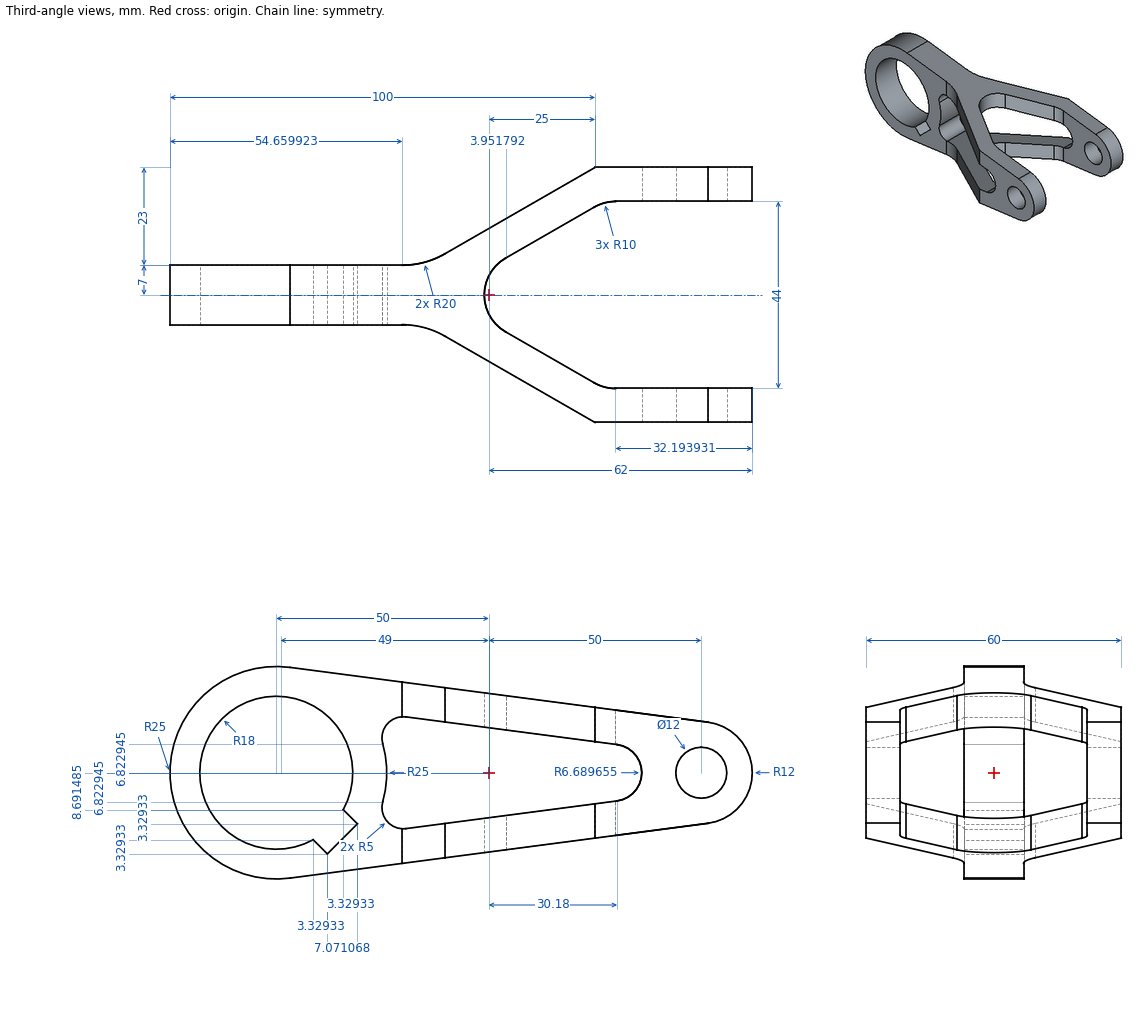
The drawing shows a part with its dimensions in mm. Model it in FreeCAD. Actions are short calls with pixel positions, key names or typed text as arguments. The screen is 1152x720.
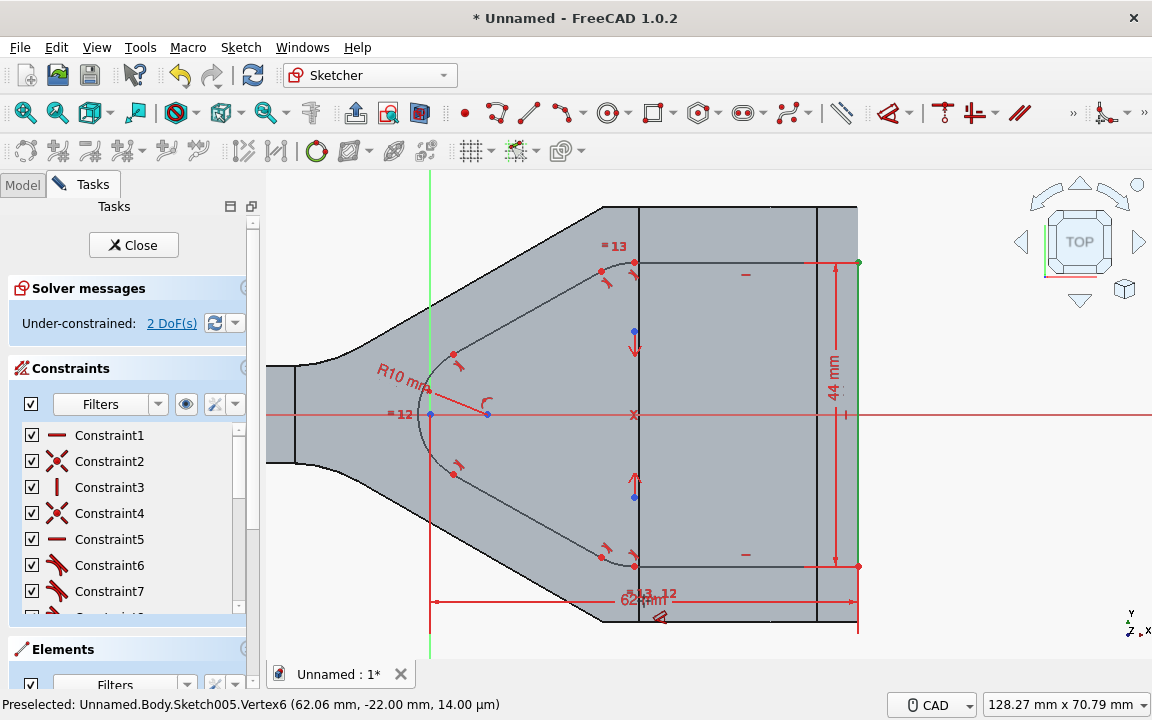
click(702, 567)
click(747, 601)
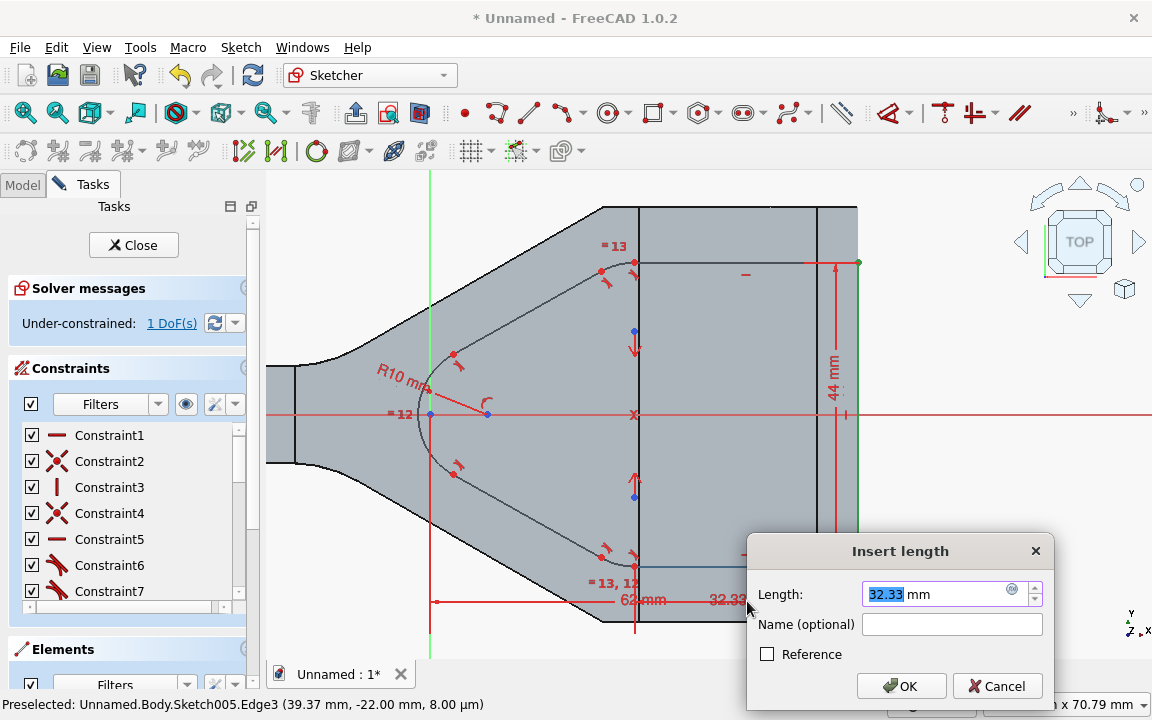
text(32.193931)
key(Return)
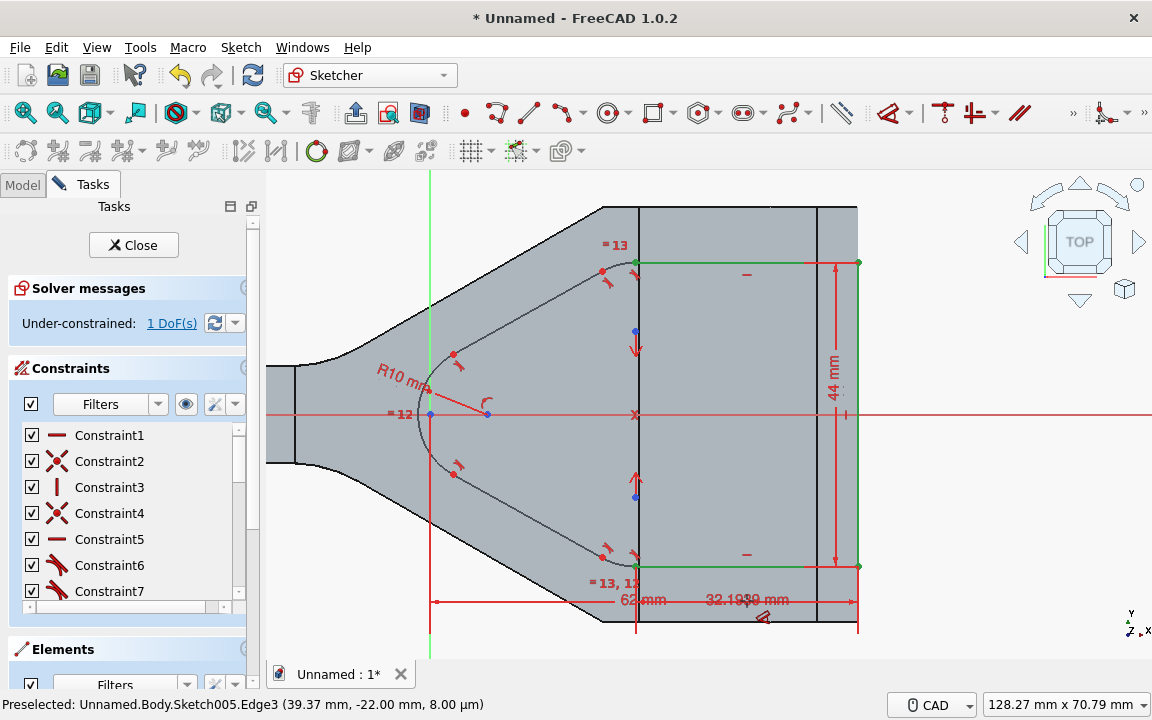
scroll(454, 354, up, 2)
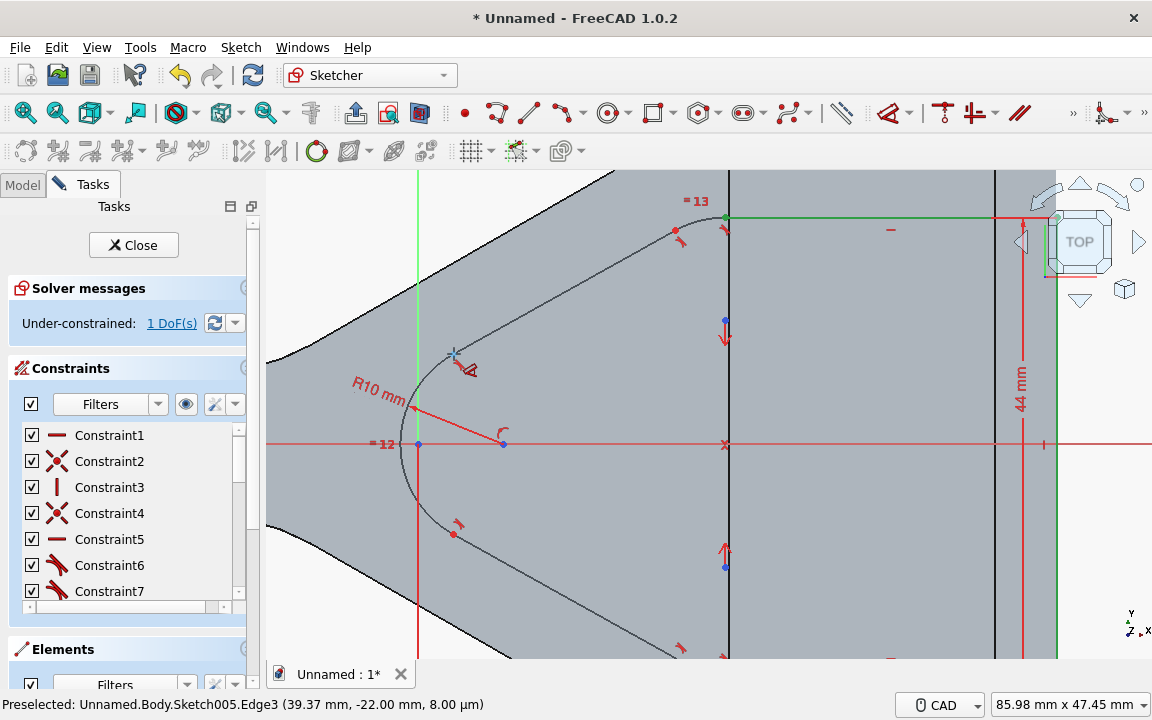
click(453, 354)
click(436, 320)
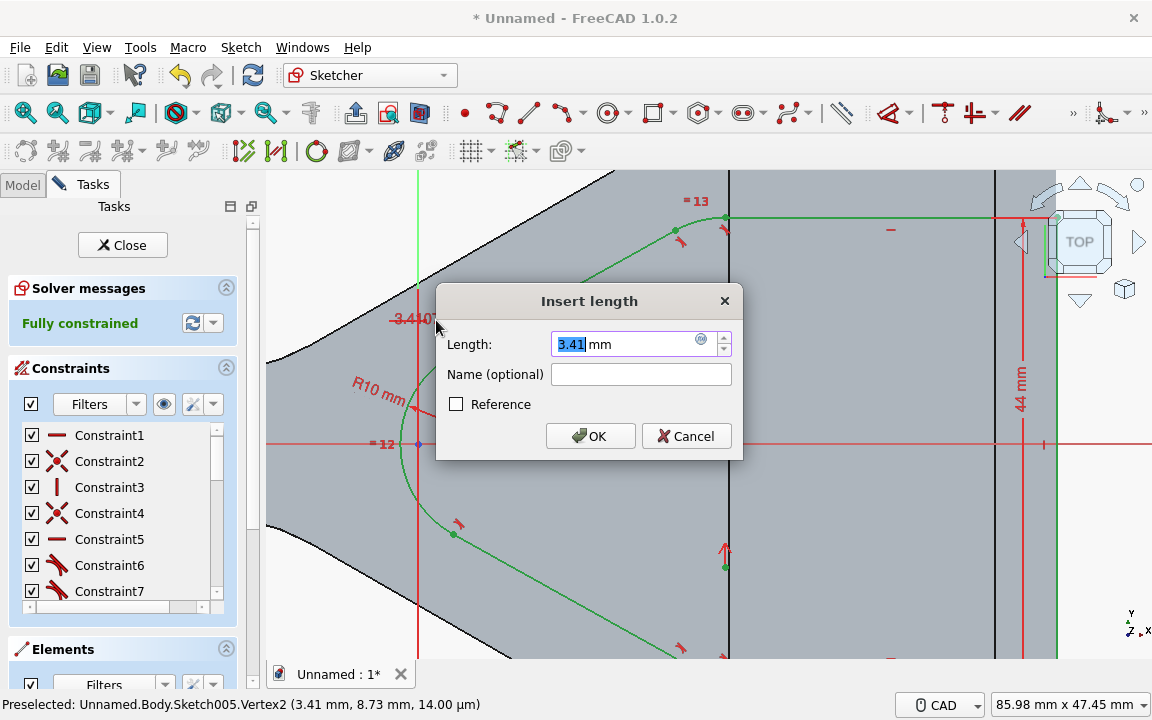
text(3.951792)
key(Return)
key(Escape)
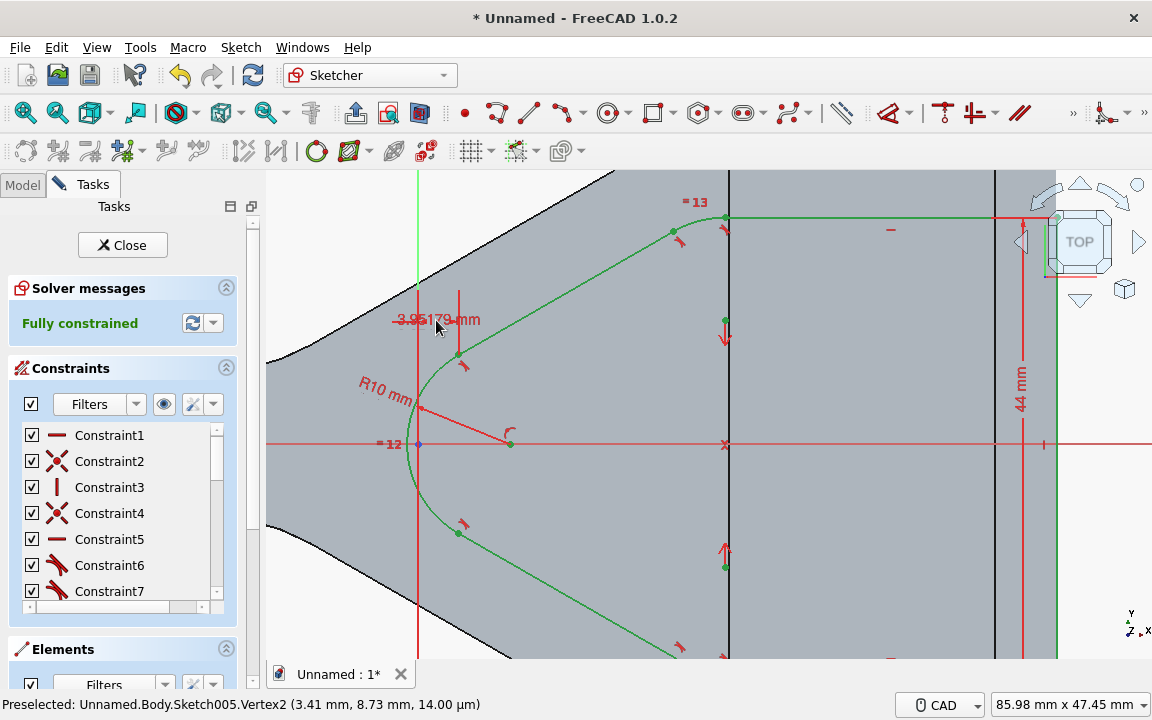
click(123, 245)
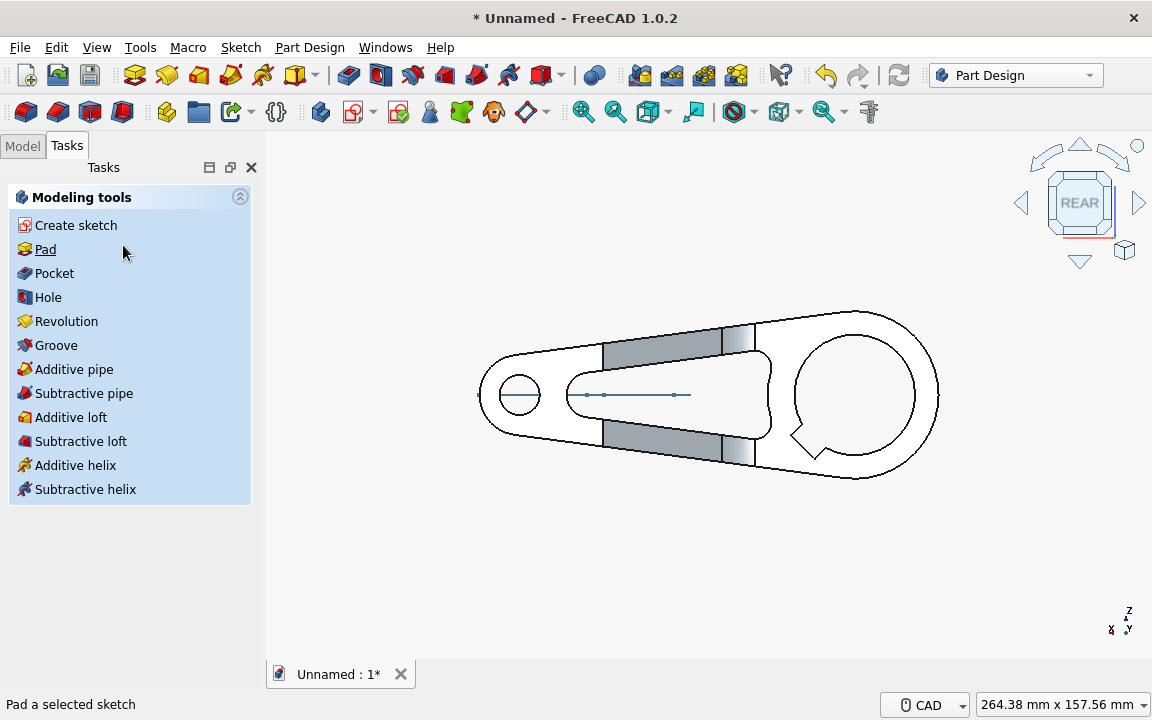
click(350, 76)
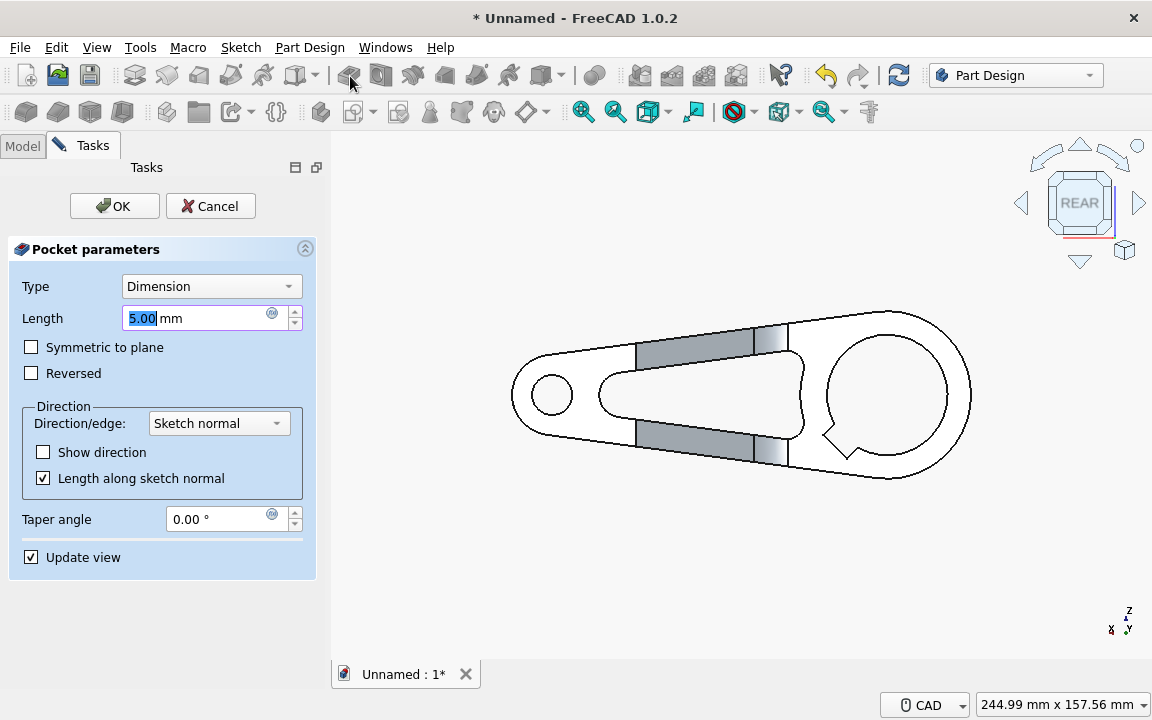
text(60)
key(Tab)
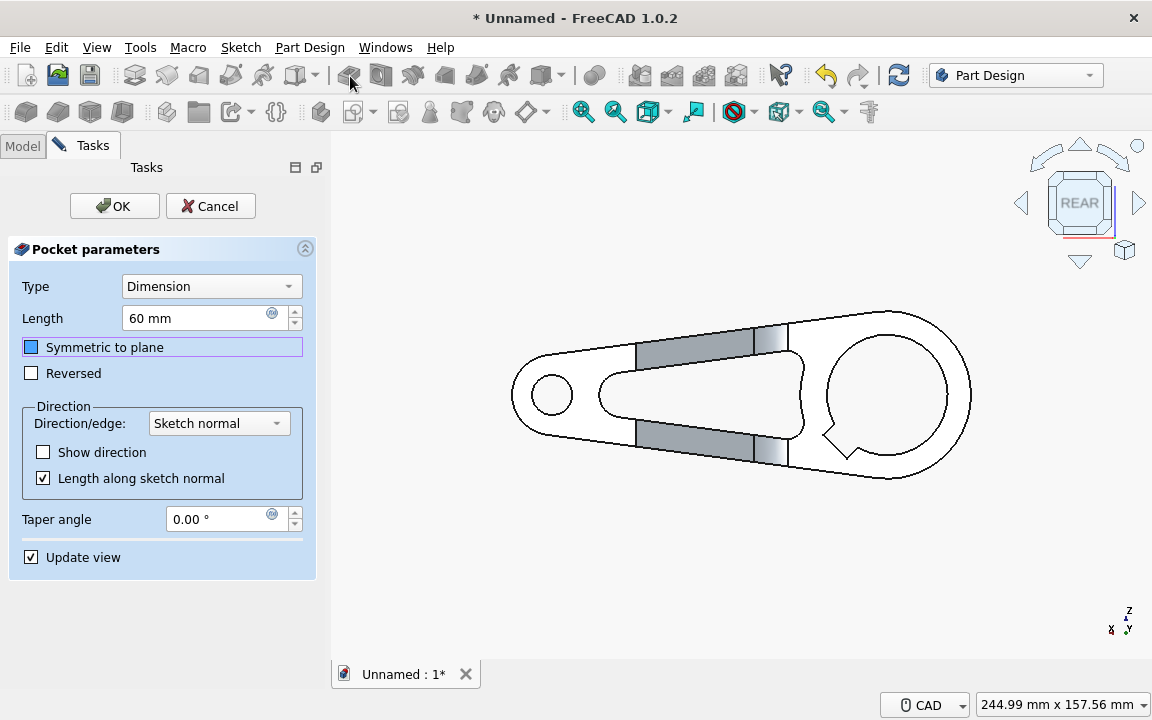
click(30, 347)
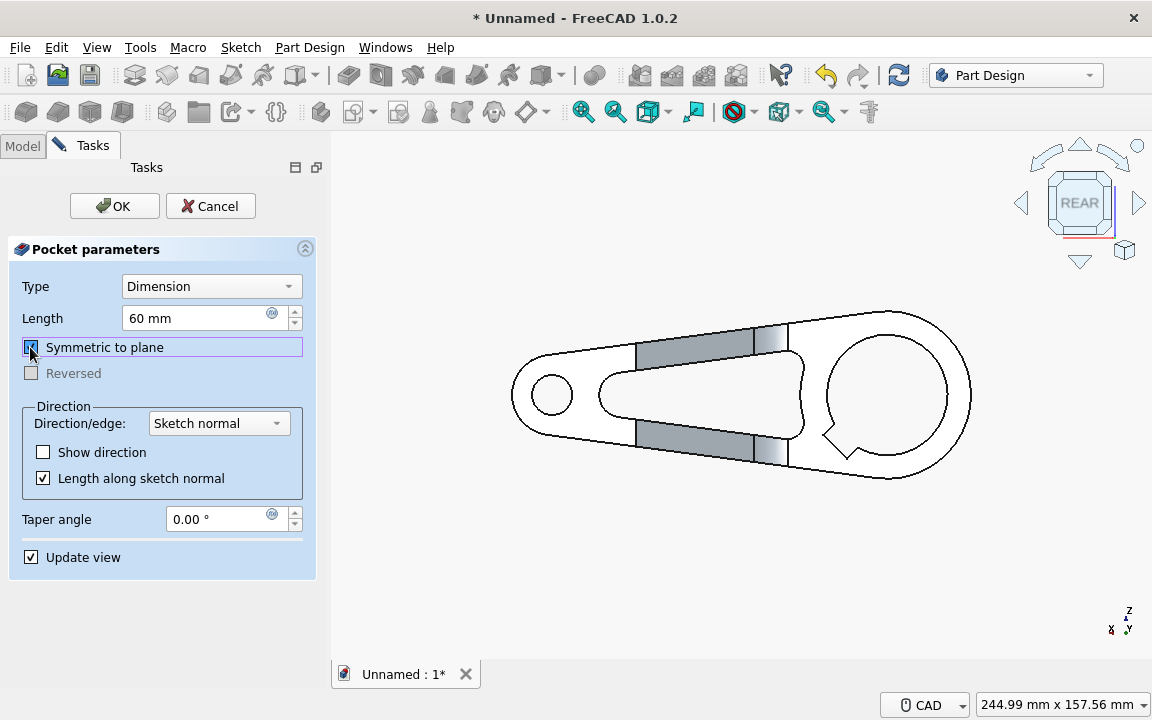
click(115, 206)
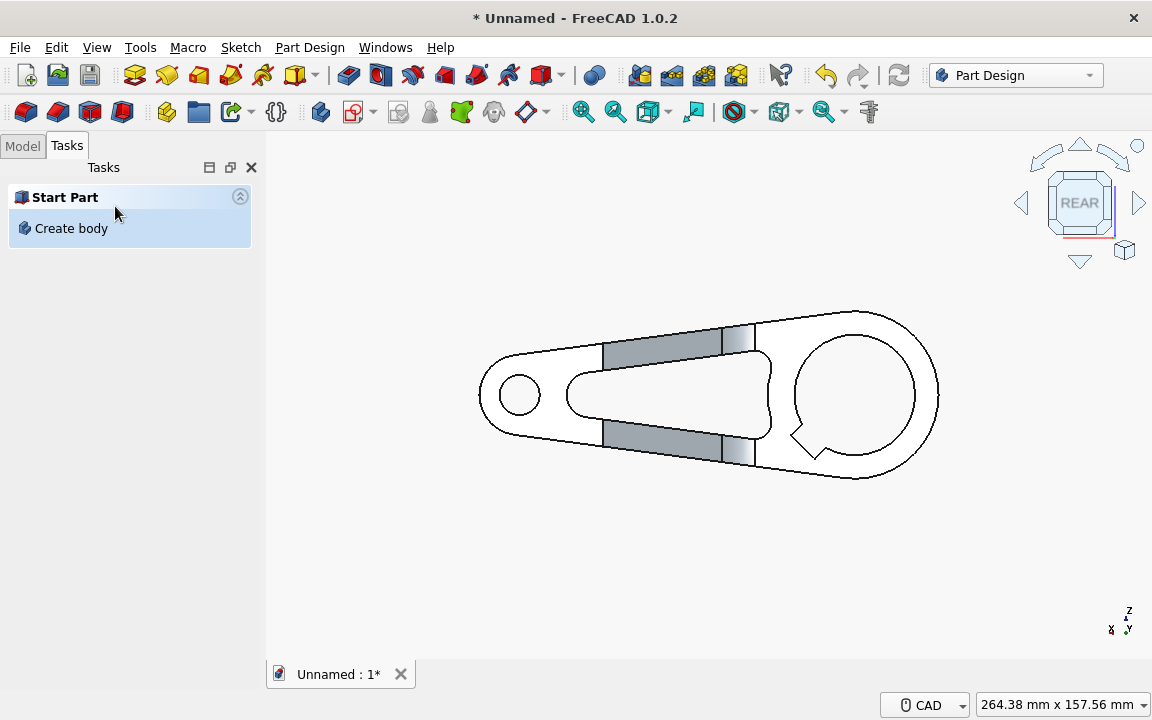
key(0)